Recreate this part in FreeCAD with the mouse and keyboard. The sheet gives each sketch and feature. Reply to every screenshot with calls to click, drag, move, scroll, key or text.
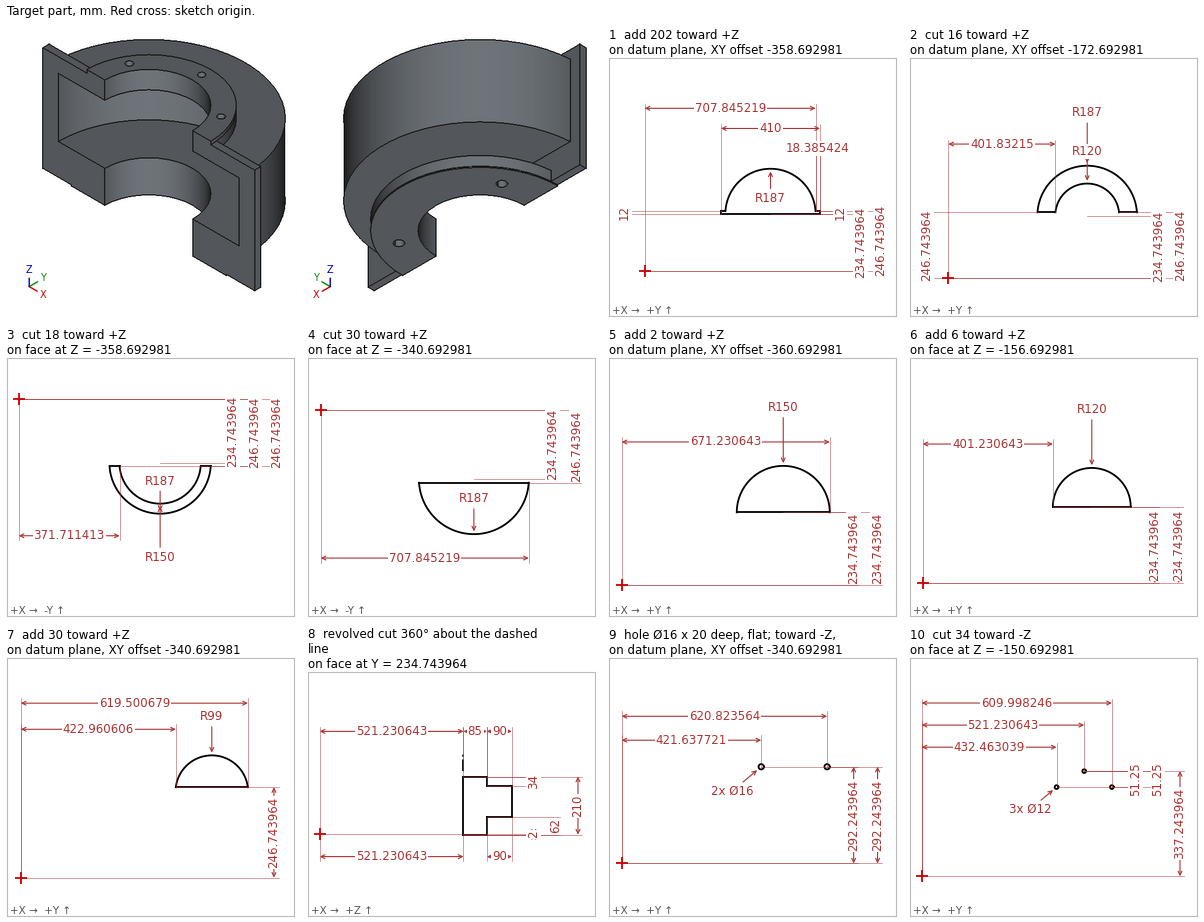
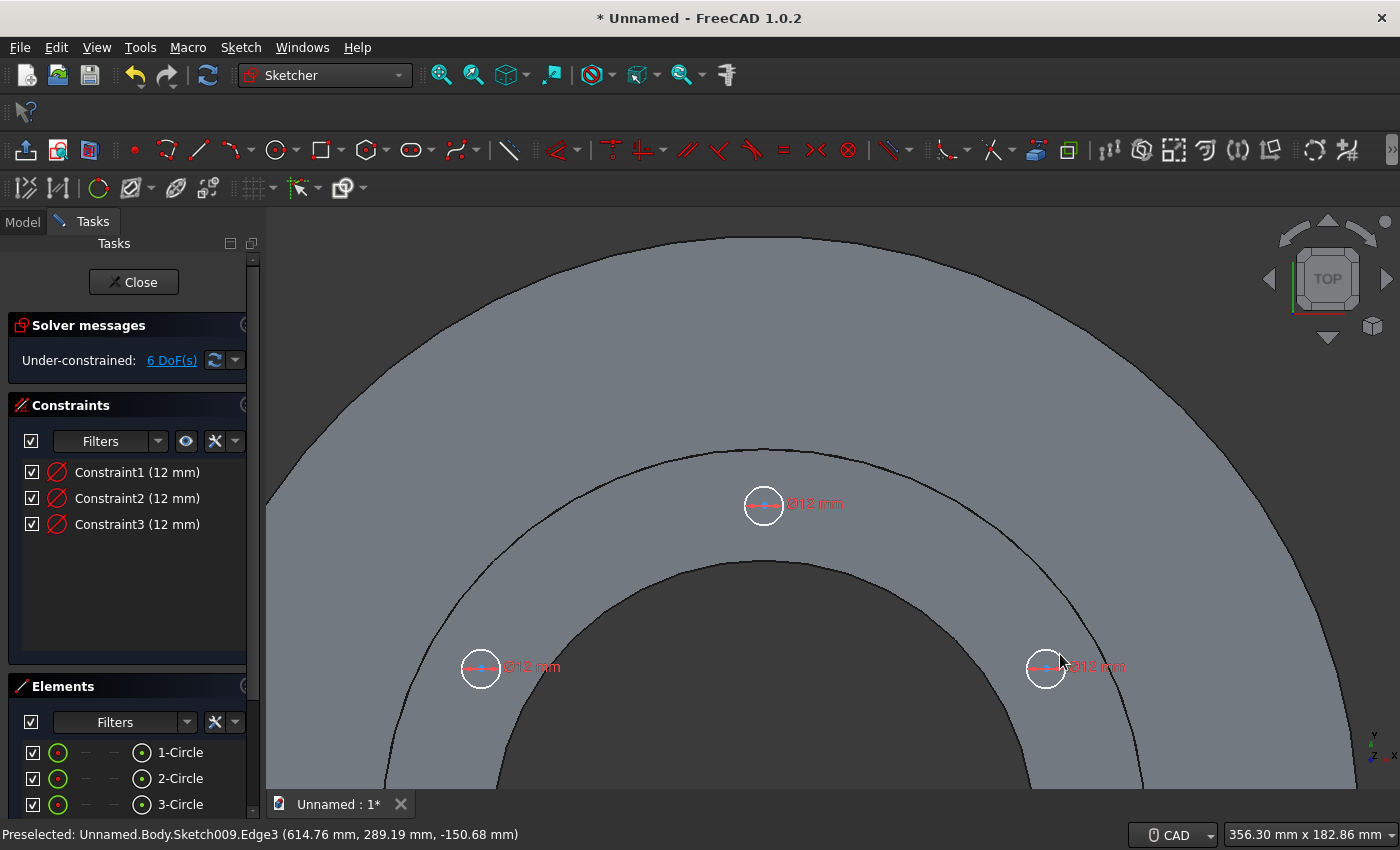
key(d)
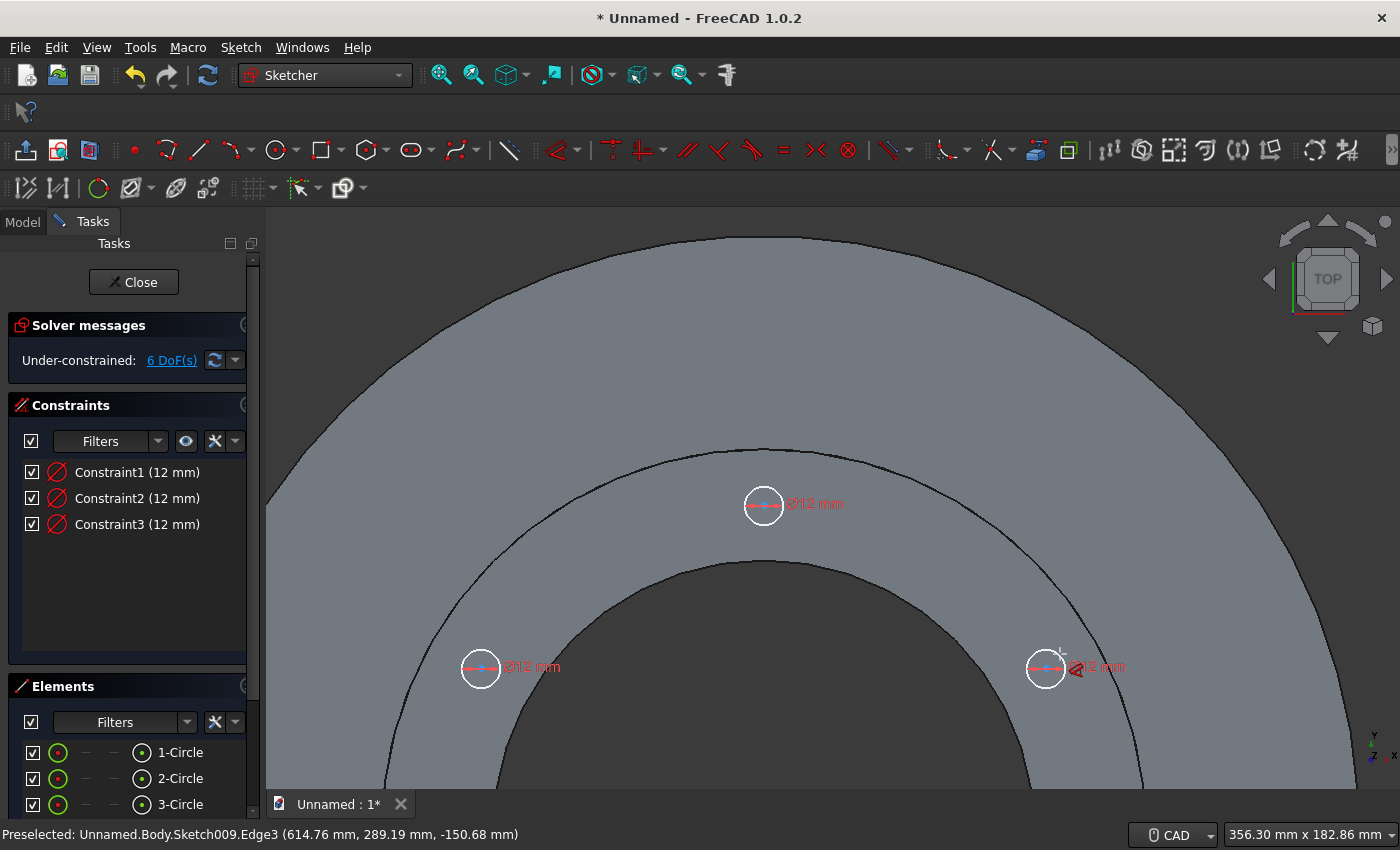
click(764, 506)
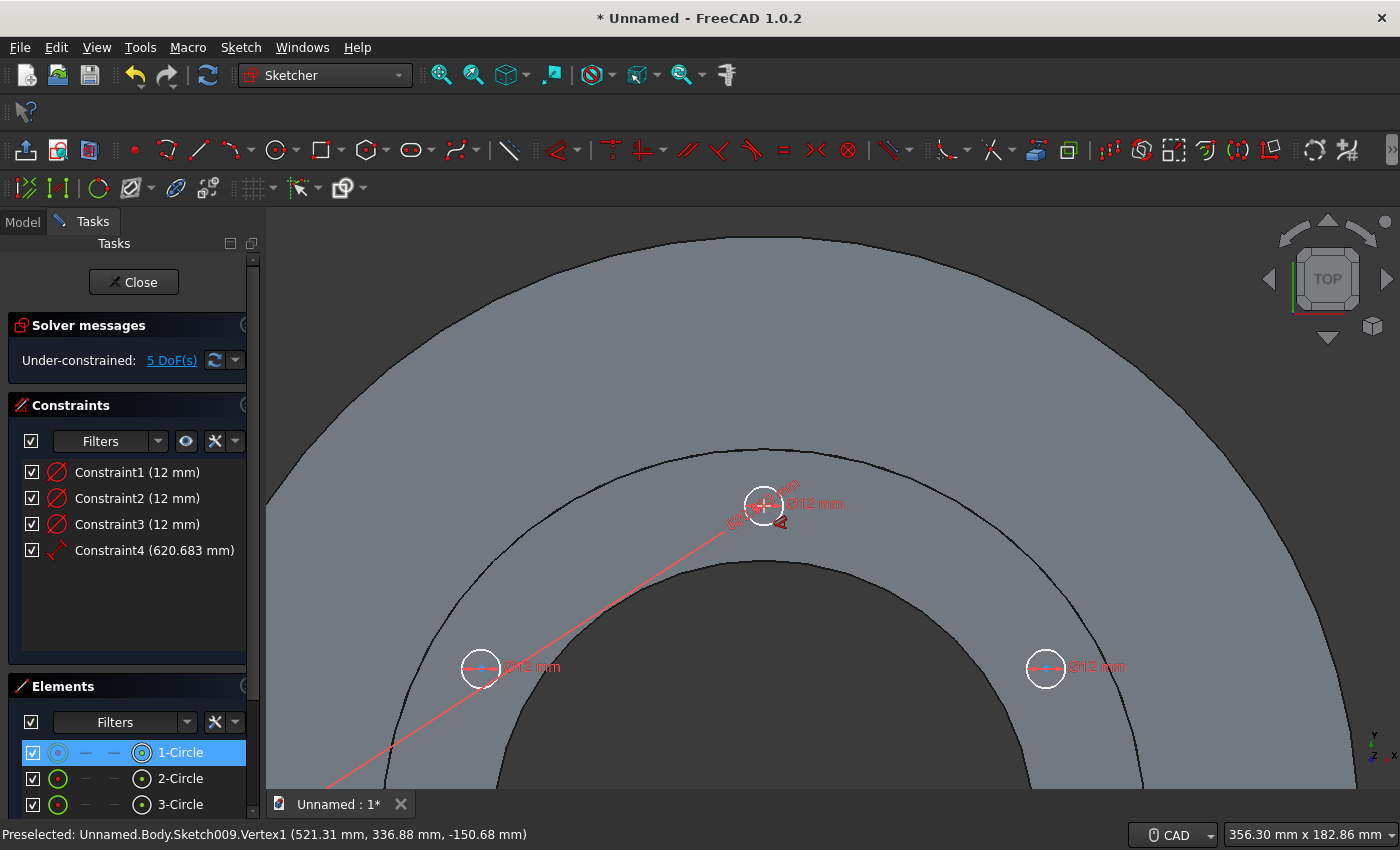
click(481, 669)
click(447, 587)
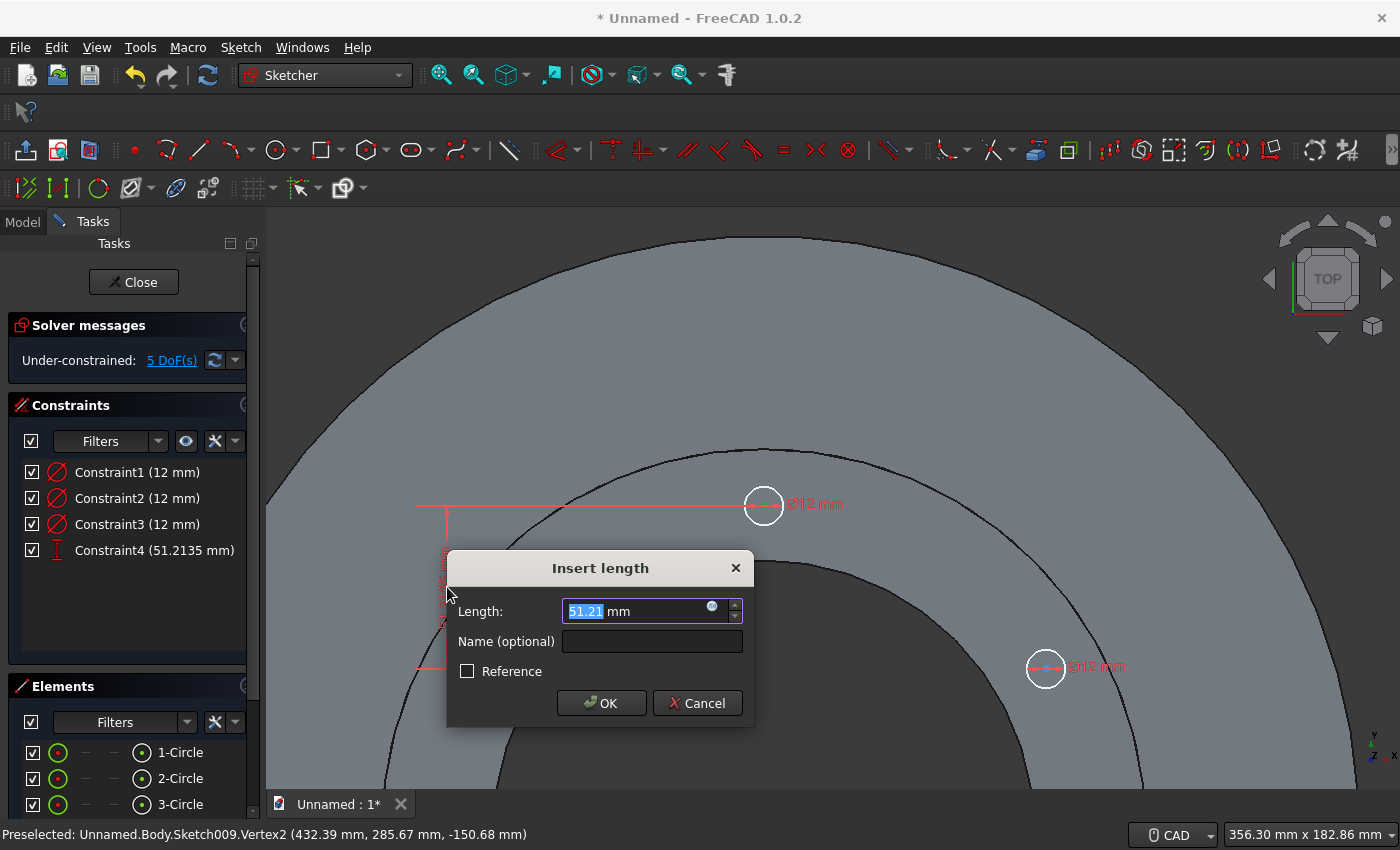
text(51.25)
key(Return)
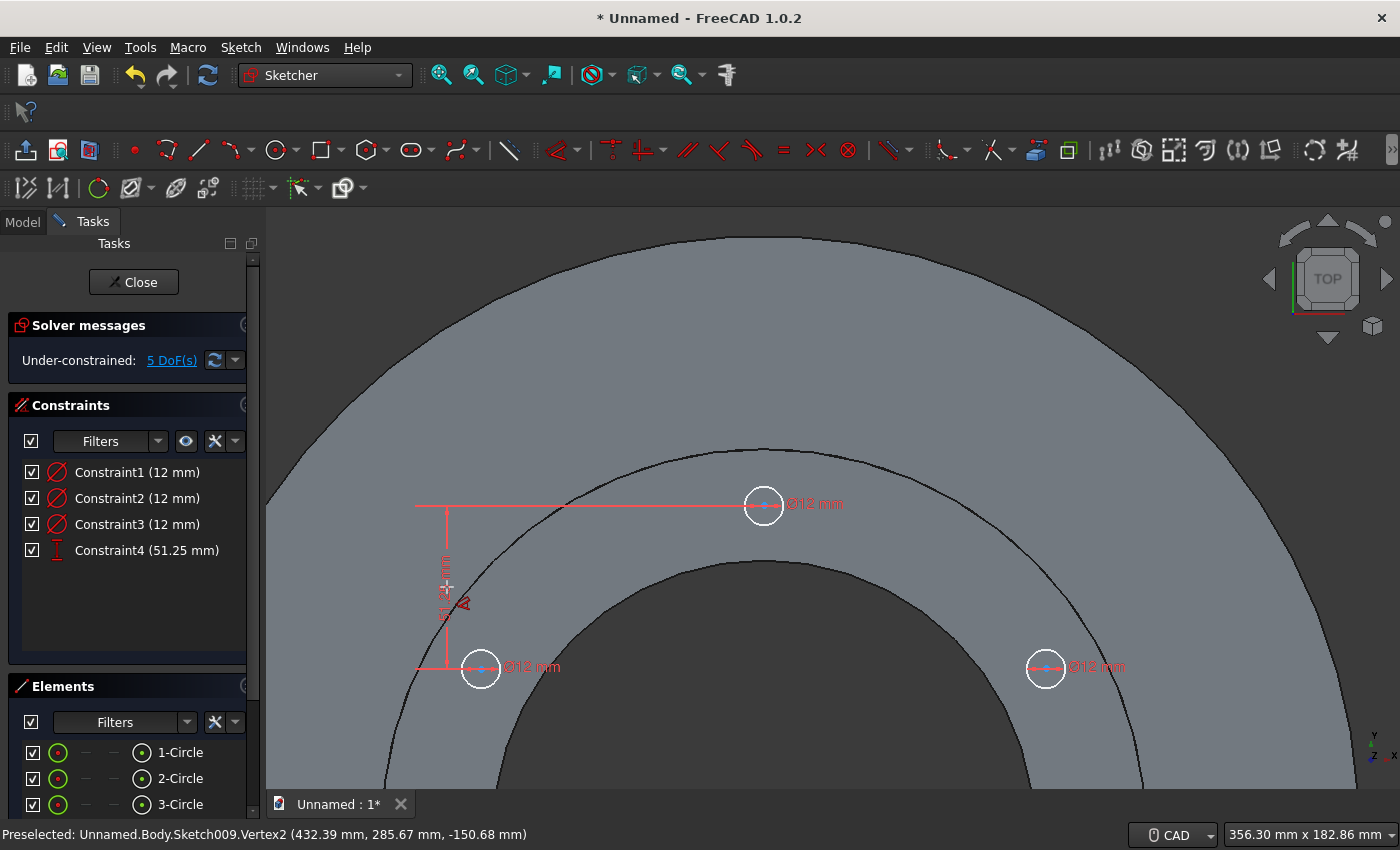
click(764, 506)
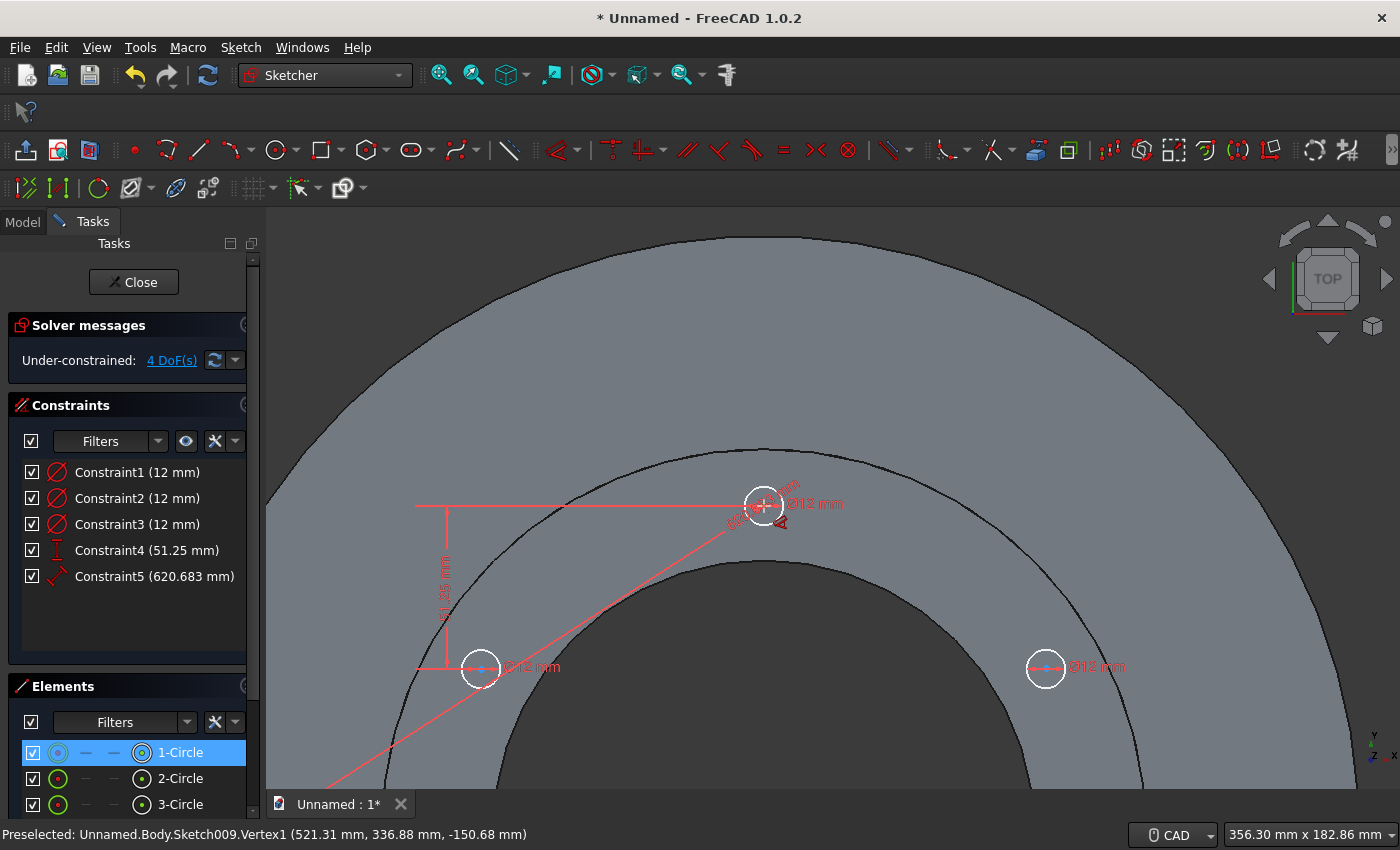
click(1046, 669)
click(1080, 587)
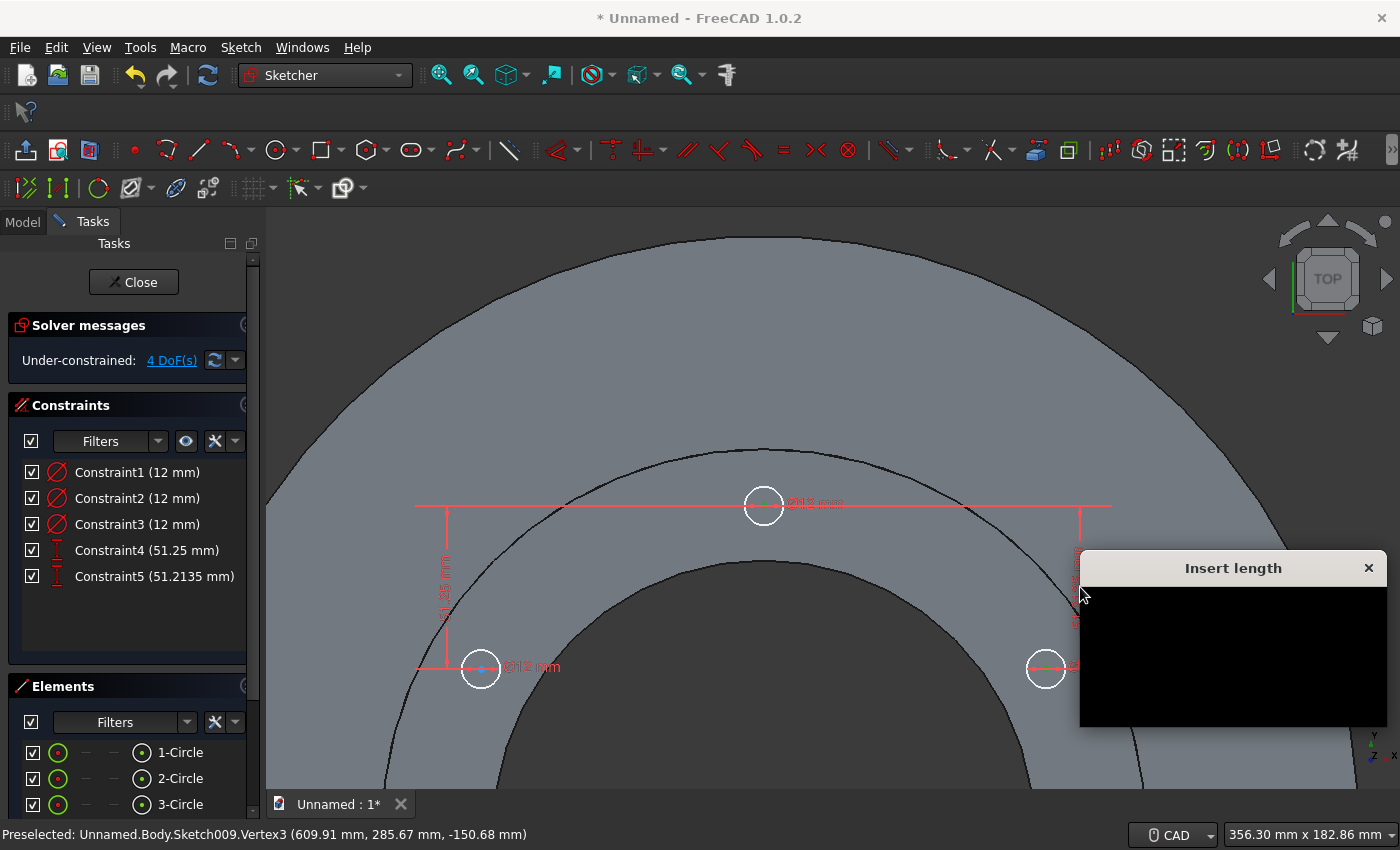
text(51.25)
key(Return)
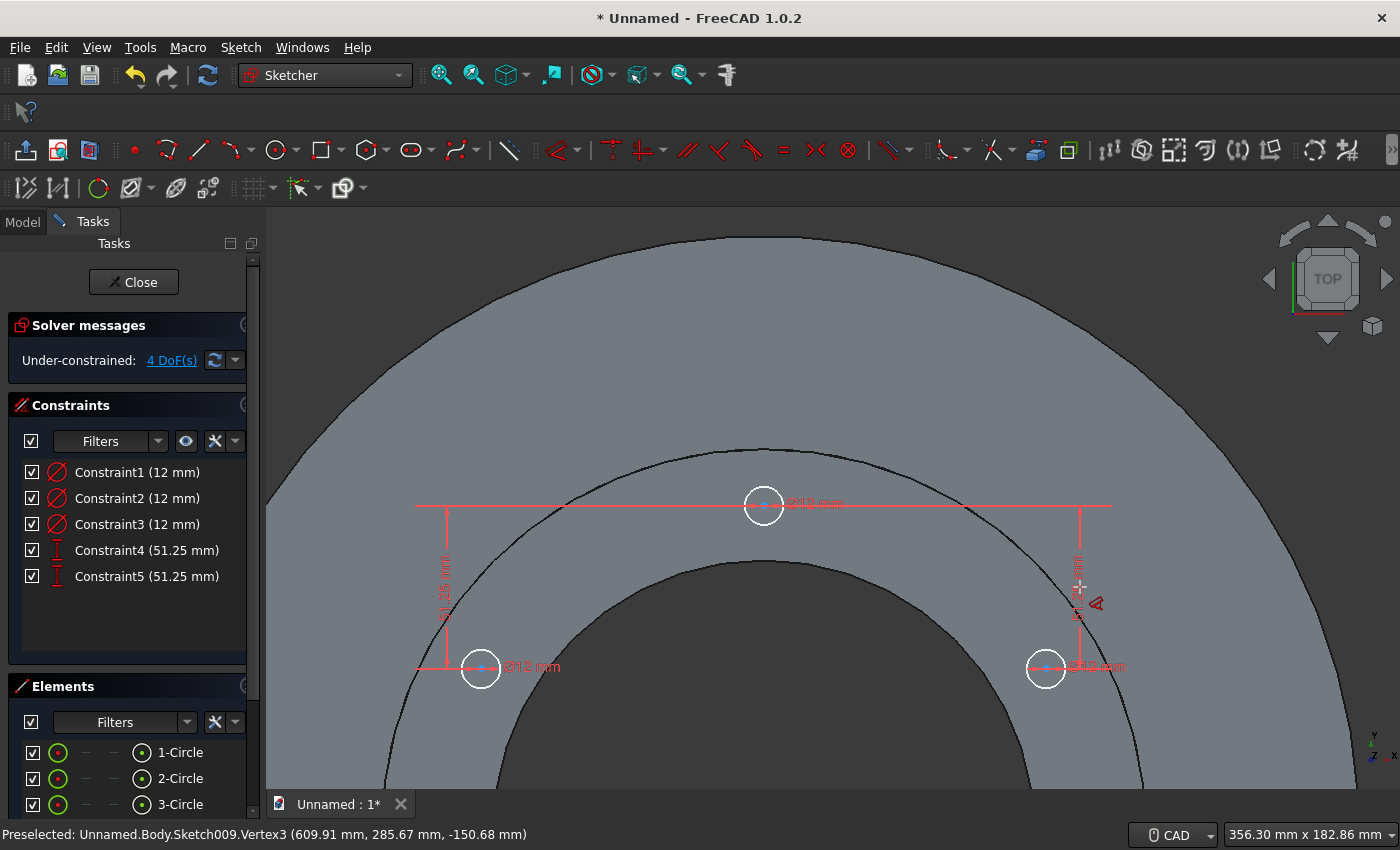
click(764, 506)
click(529, 472)